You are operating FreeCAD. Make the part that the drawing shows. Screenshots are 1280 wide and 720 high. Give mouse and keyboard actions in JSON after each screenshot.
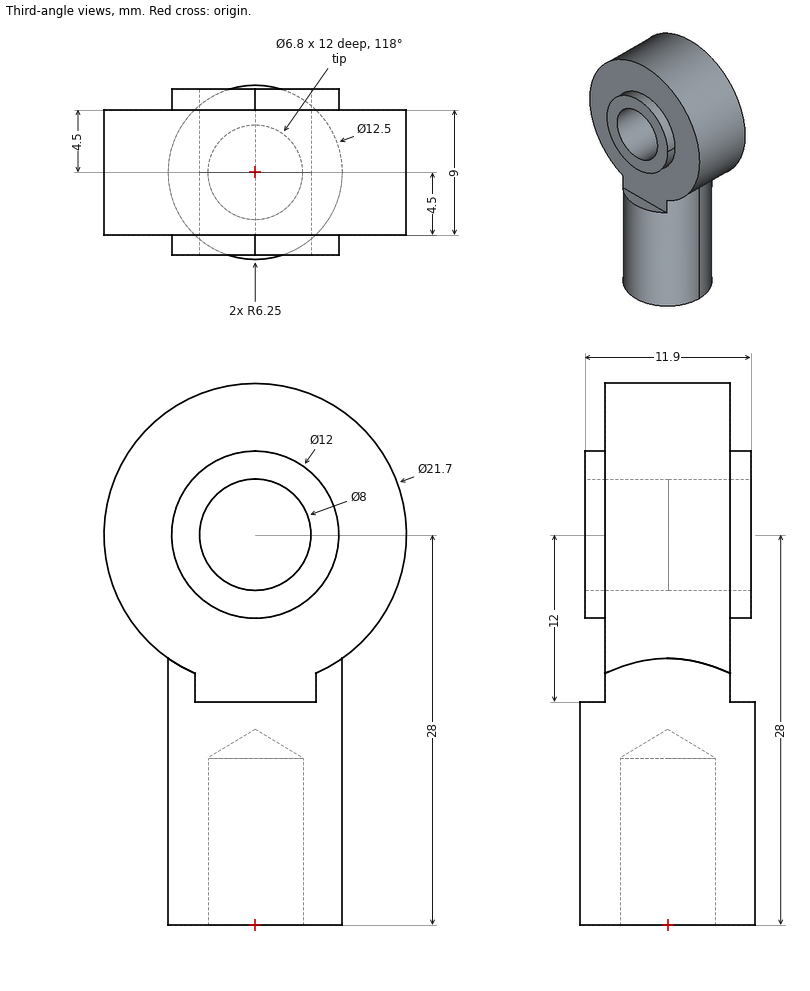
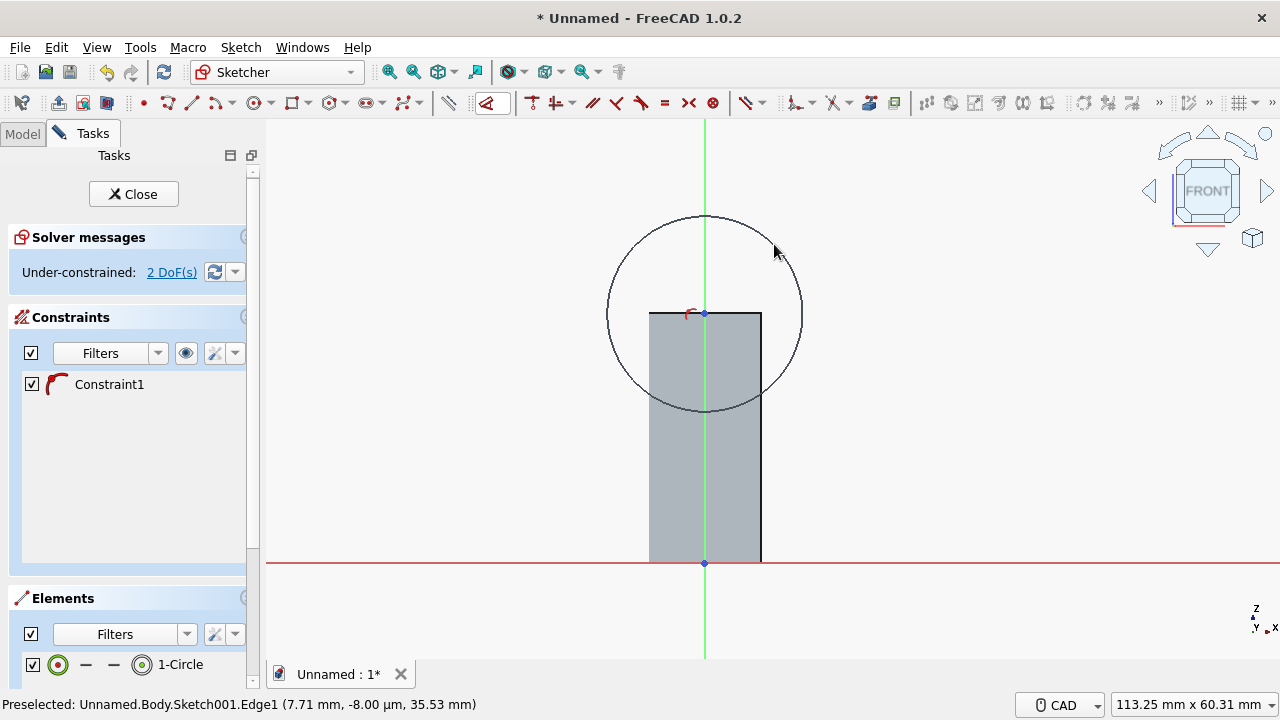
{"action": "left_click", "coordinate": [774, 245]}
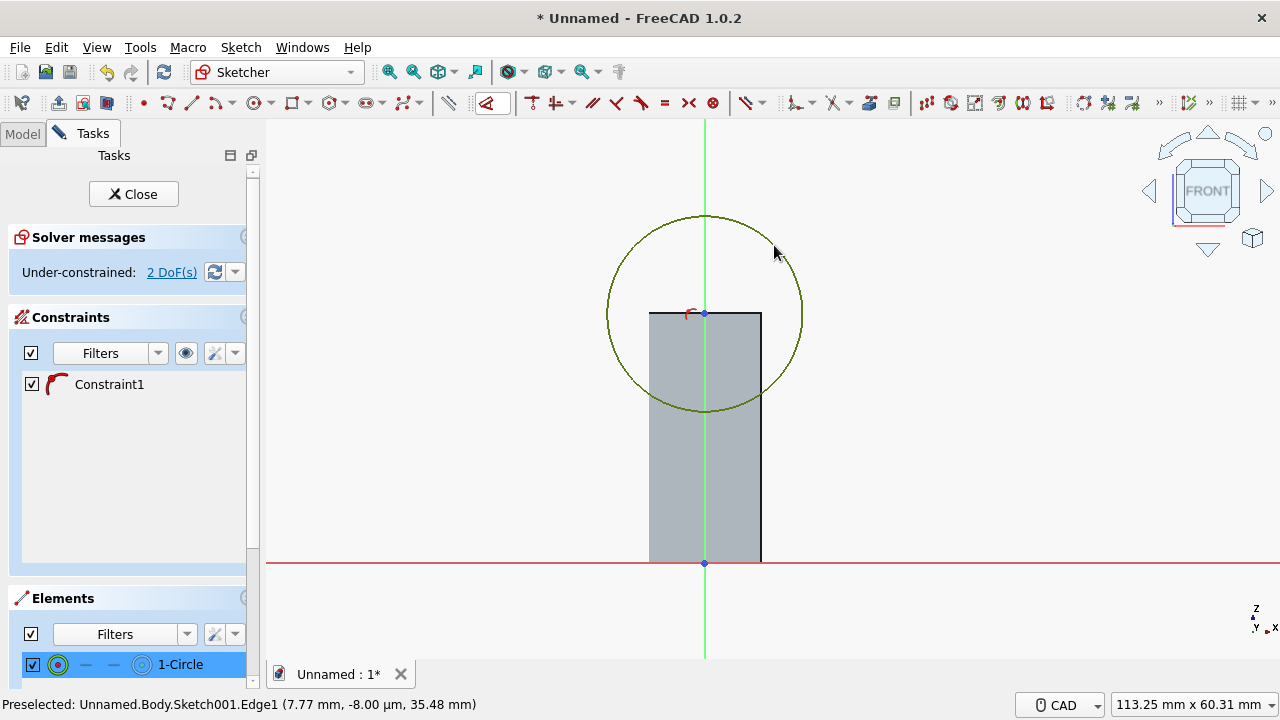
{"action": "key", "text": "k o"}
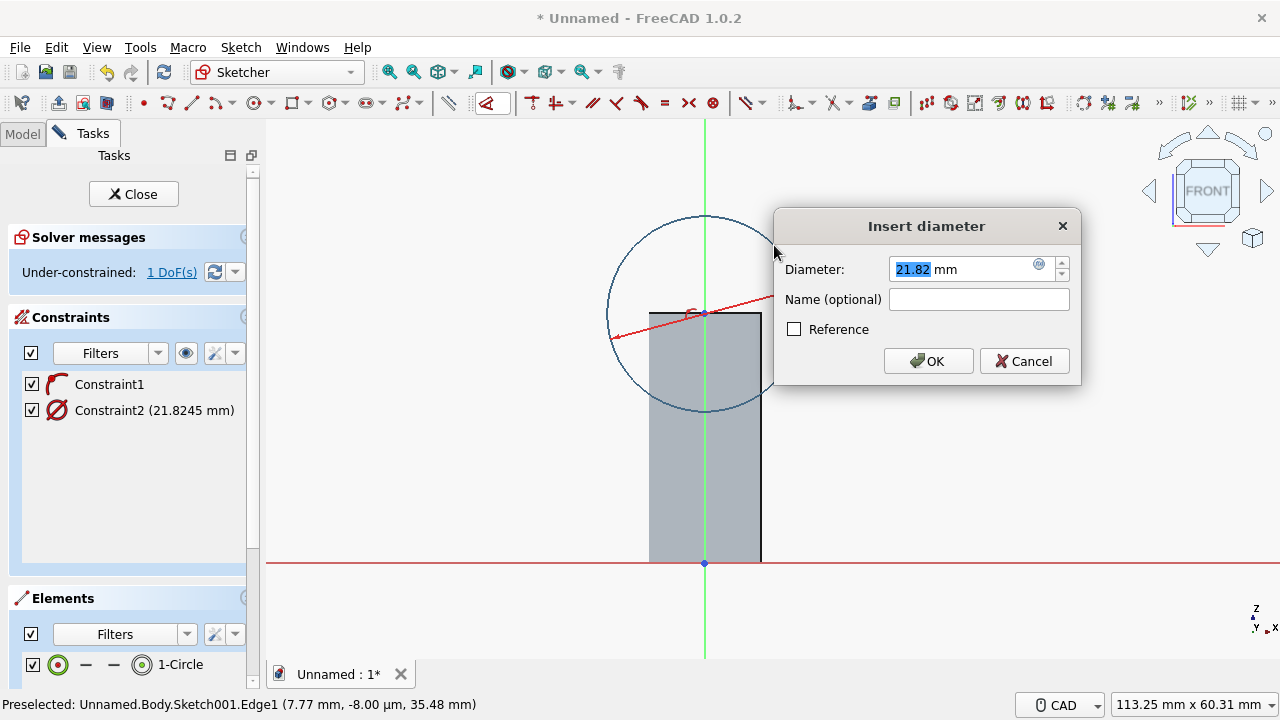
{"action": "type", "text": "21.7"}
{"action": "key", "text": "Return"}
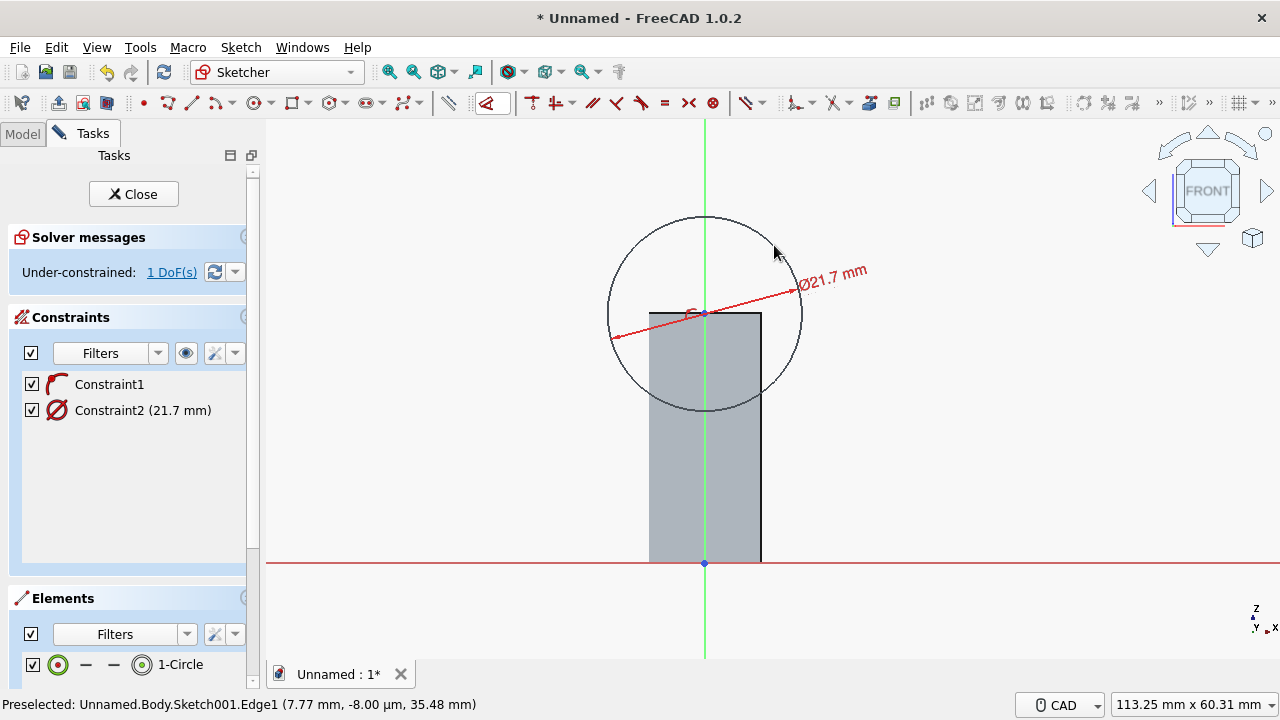
{"action": "left_click", "coordinate": [705, 314]}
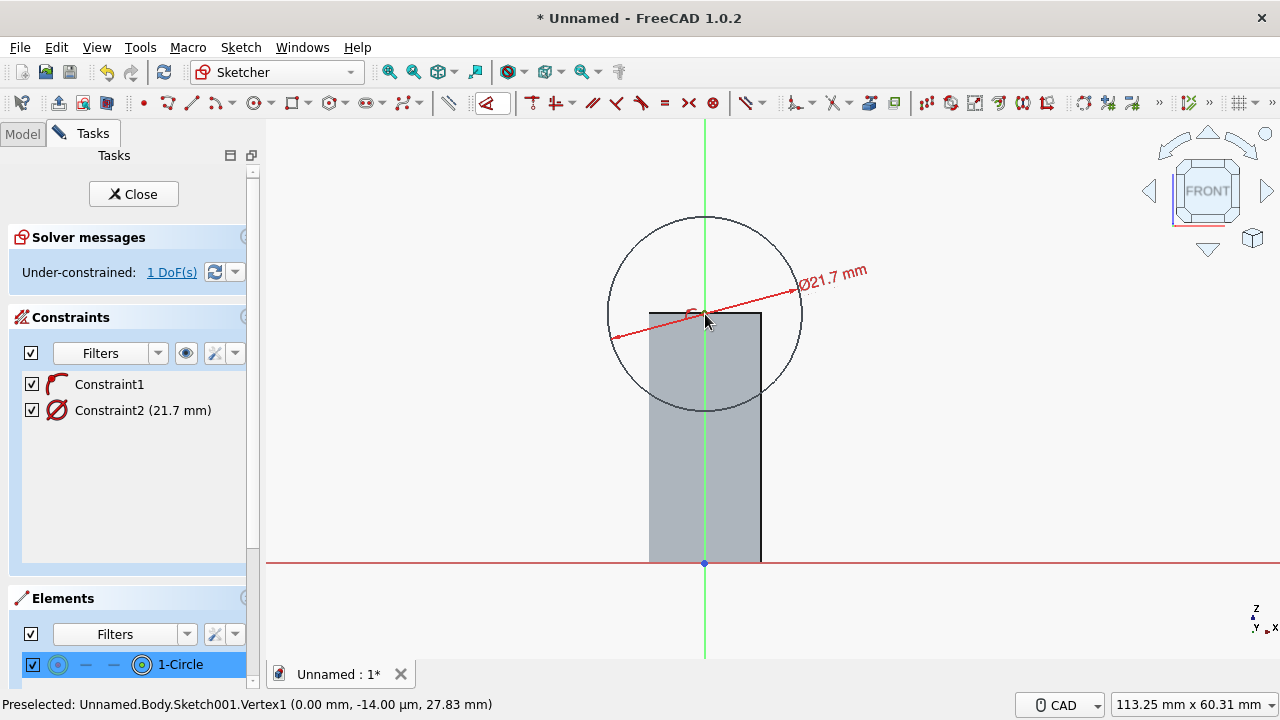
{"action": "key", "text": "i"}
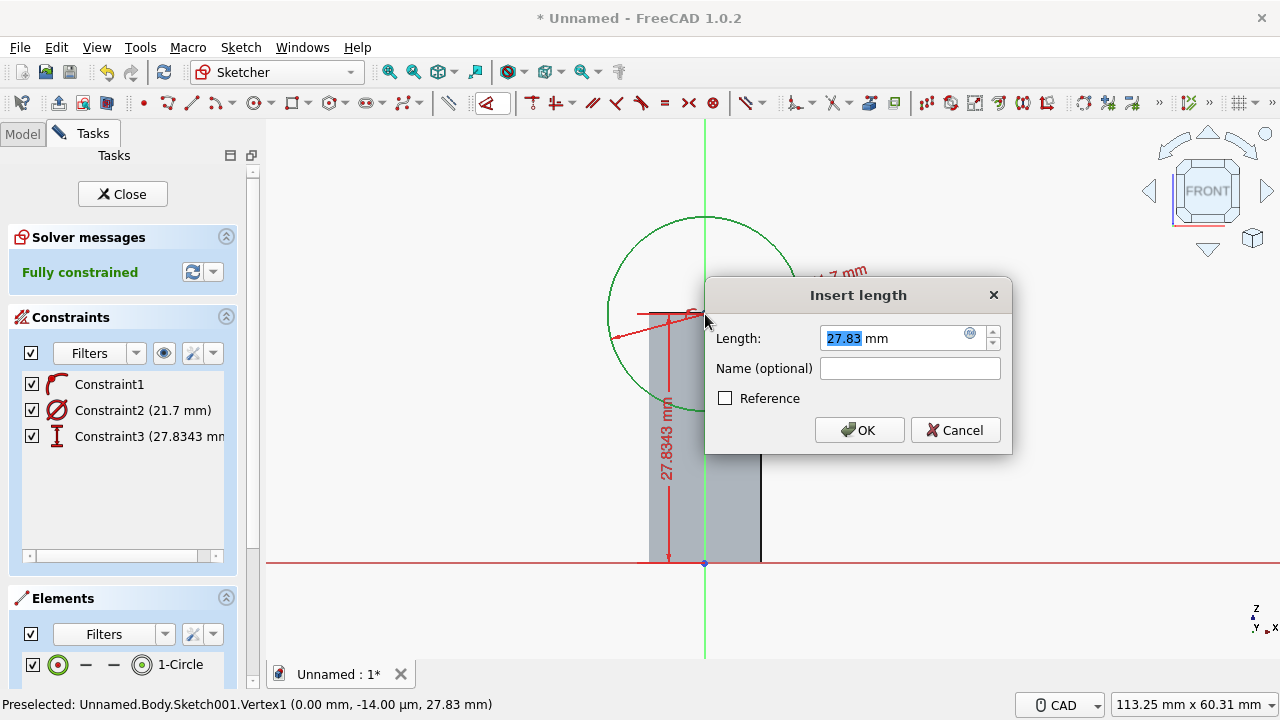
{"action": "type", "text": "28"}
{"action": "key", "text": "Return"}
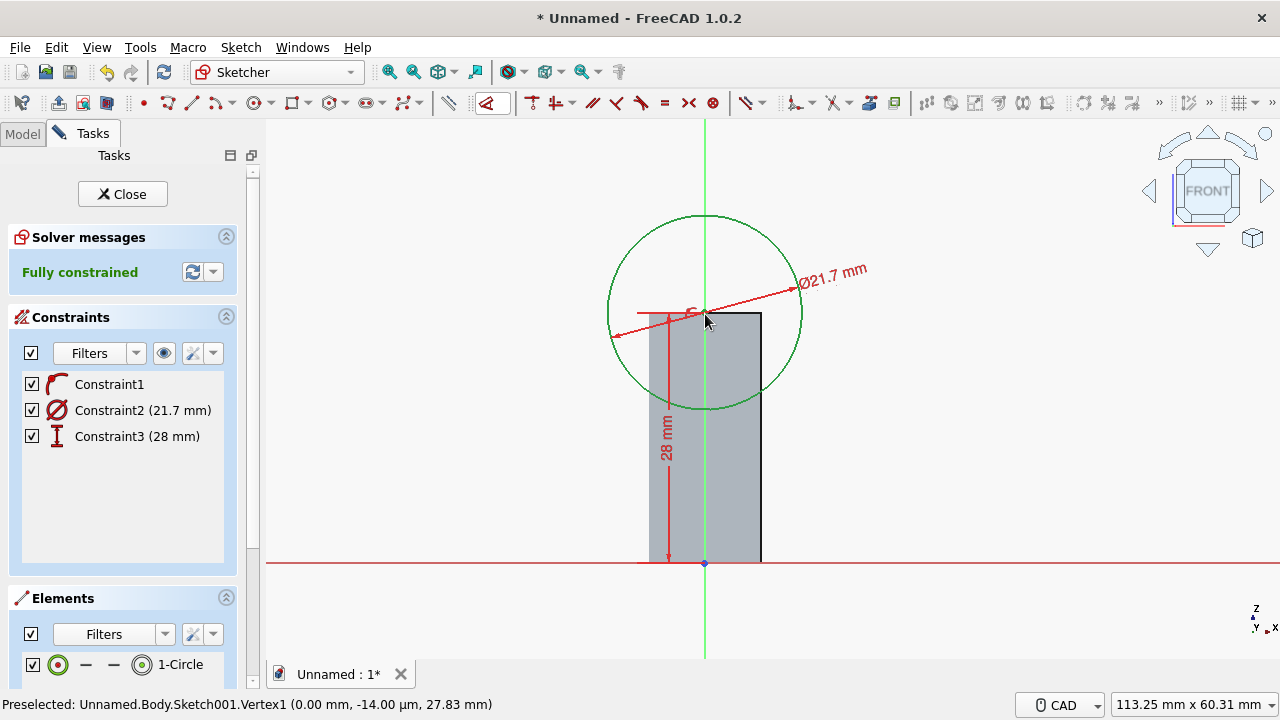
{"action": "left_click", "coordinate": [123, 194]}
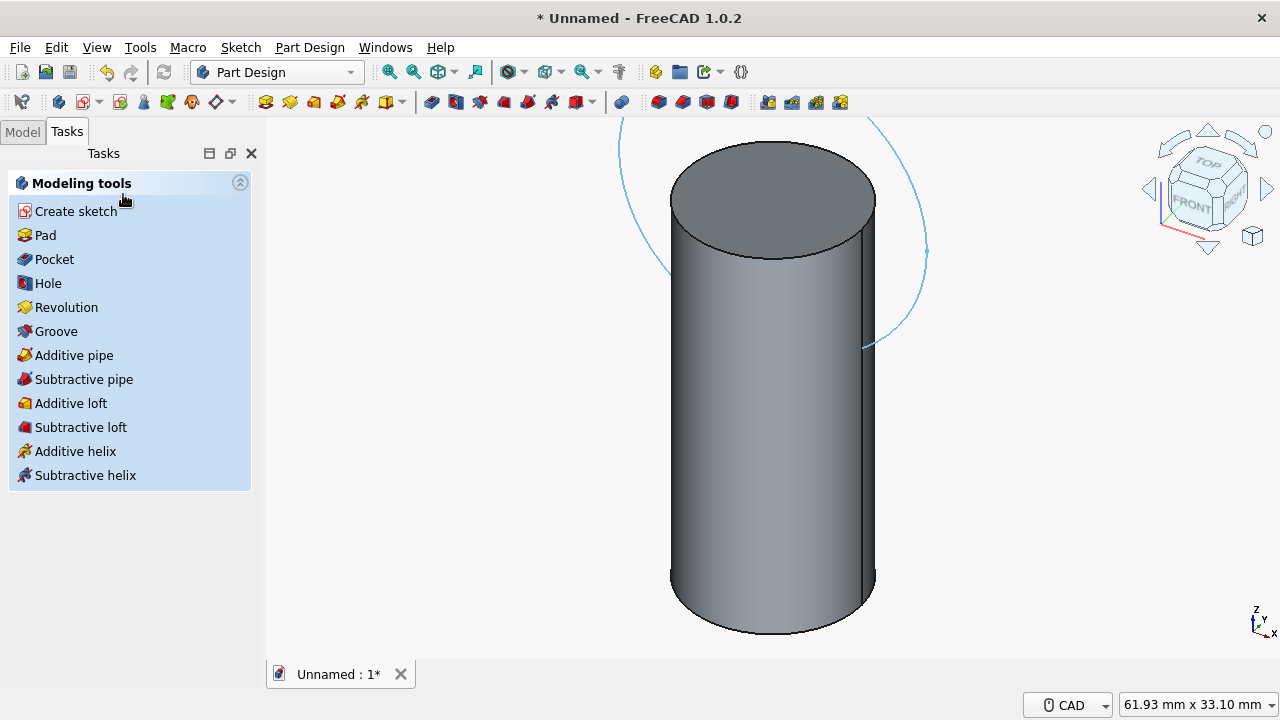
{"action": "left_click", "coordinate": [266, 102]}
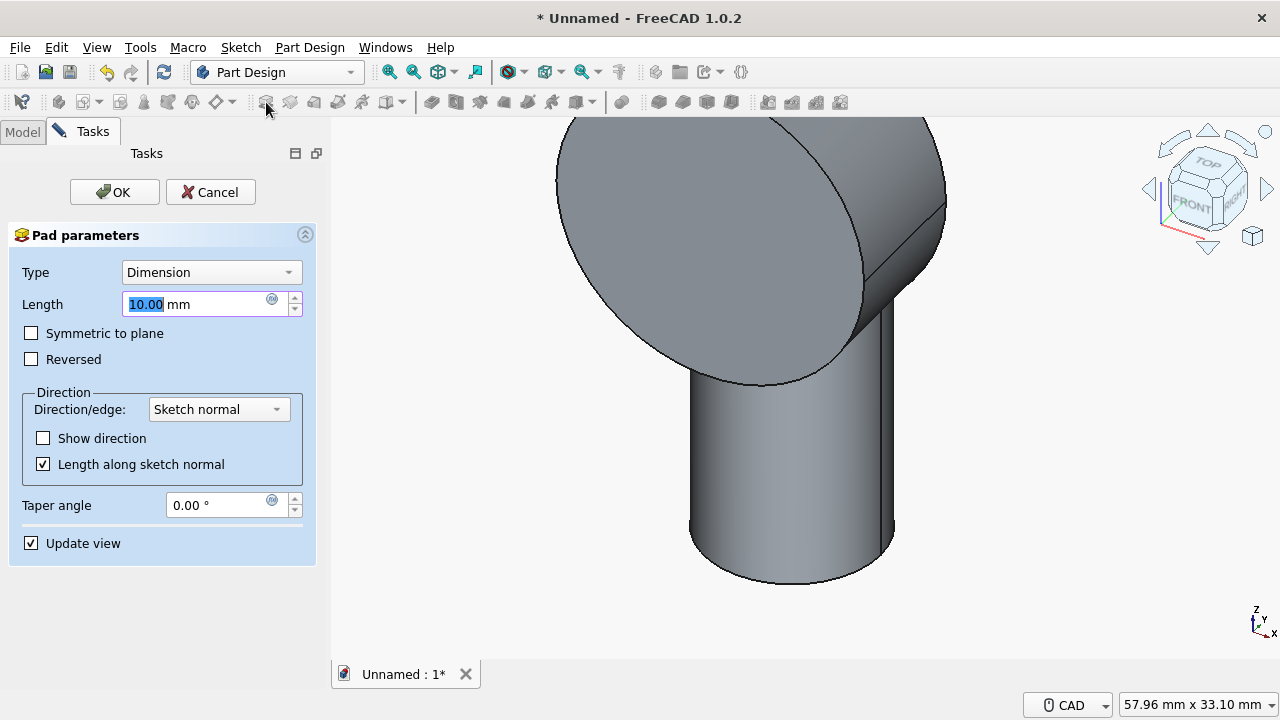
{"action": "type", "text": "9"}
{"action": "key", "text": "Tab"}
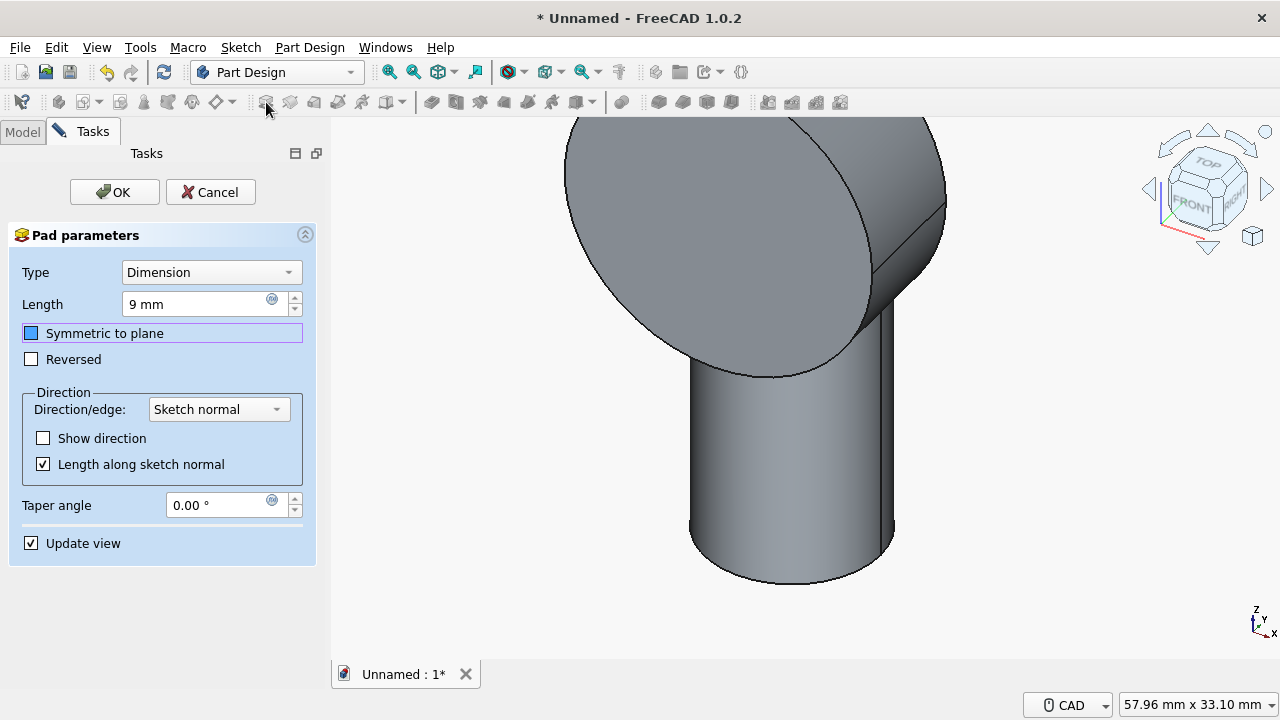
{"action": "left_click", "coordinate": [30, 333]}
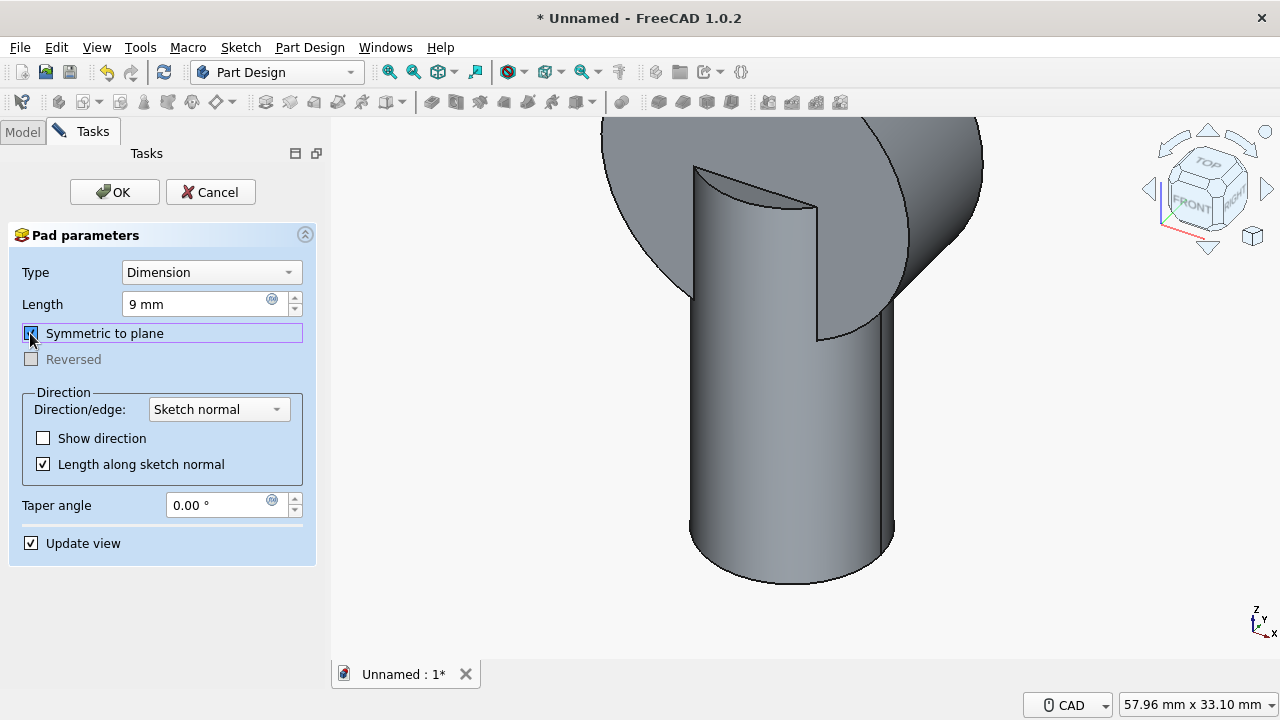
{"action": "left_click", "coordinate": [115, 192]}